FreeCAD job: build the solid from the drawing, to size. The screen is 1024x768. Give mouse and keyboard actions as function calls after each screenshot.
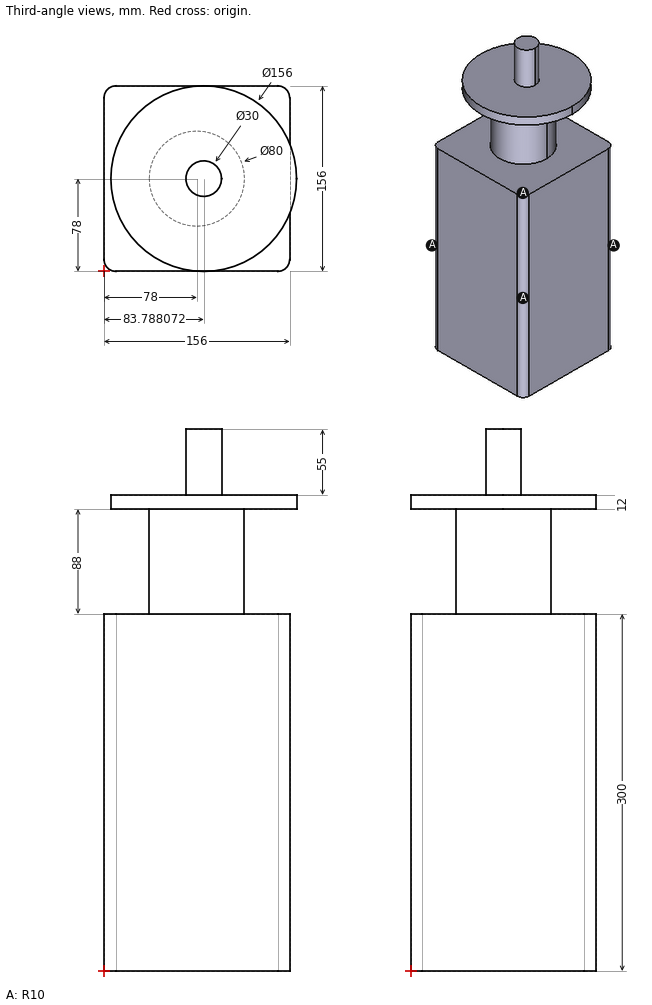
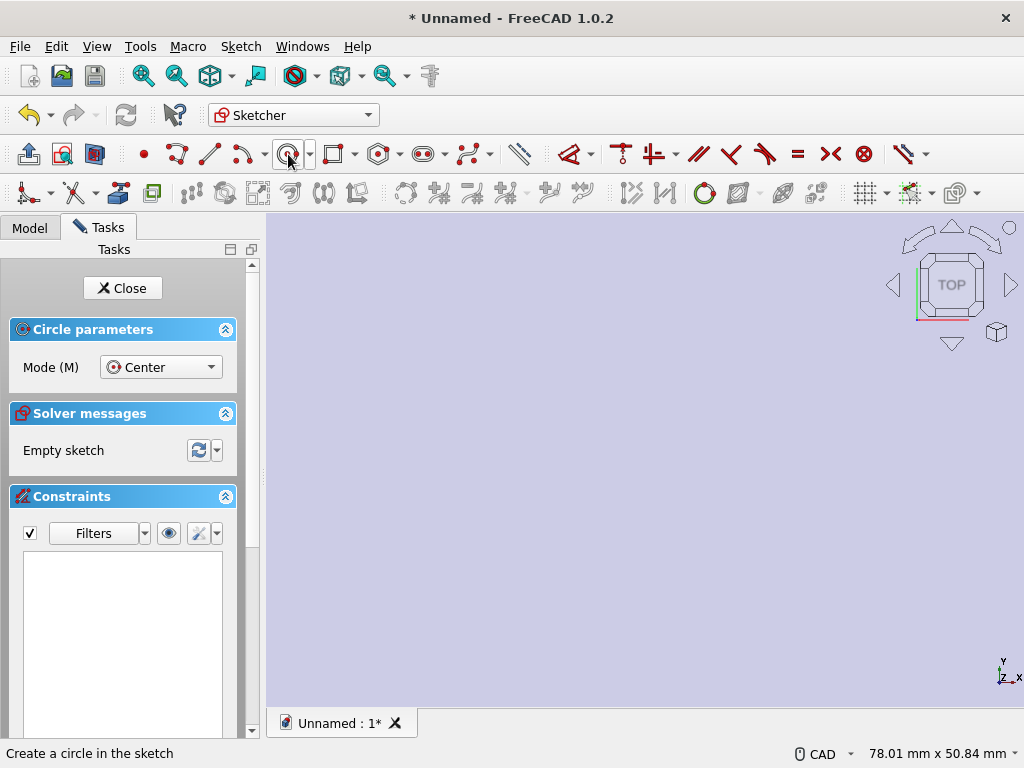
click(573, 456)
move(676, 353)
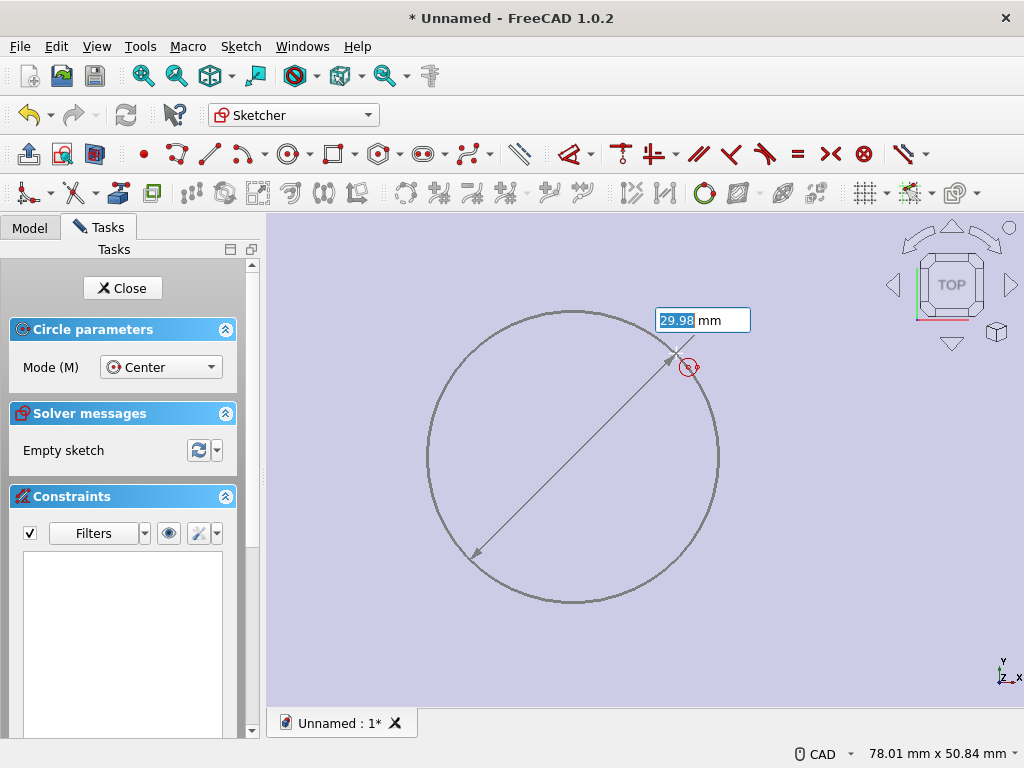
text(30)
key(Return)
key(Escape)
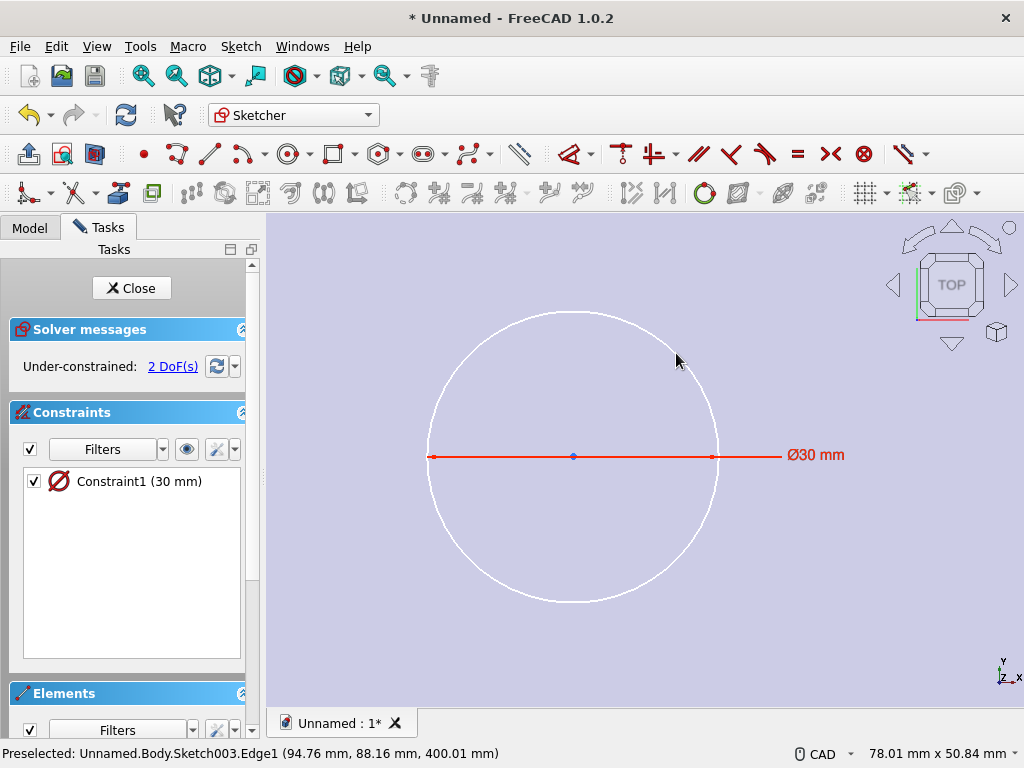
click(568, 154)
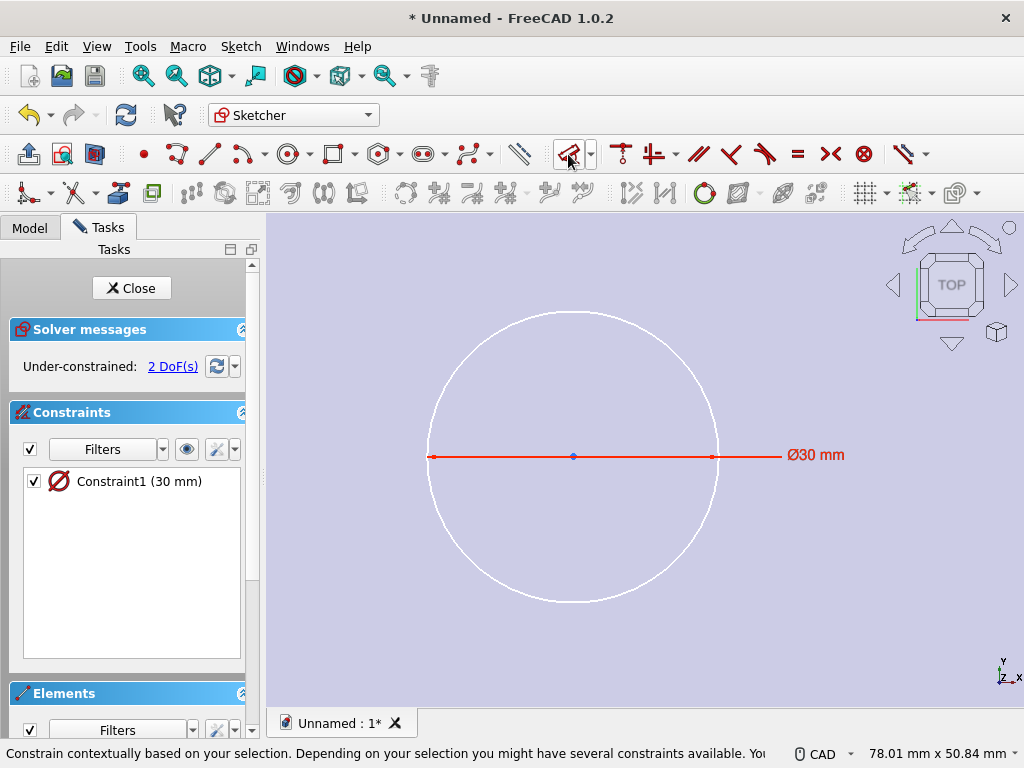
click(573, 457)
click(607, 568)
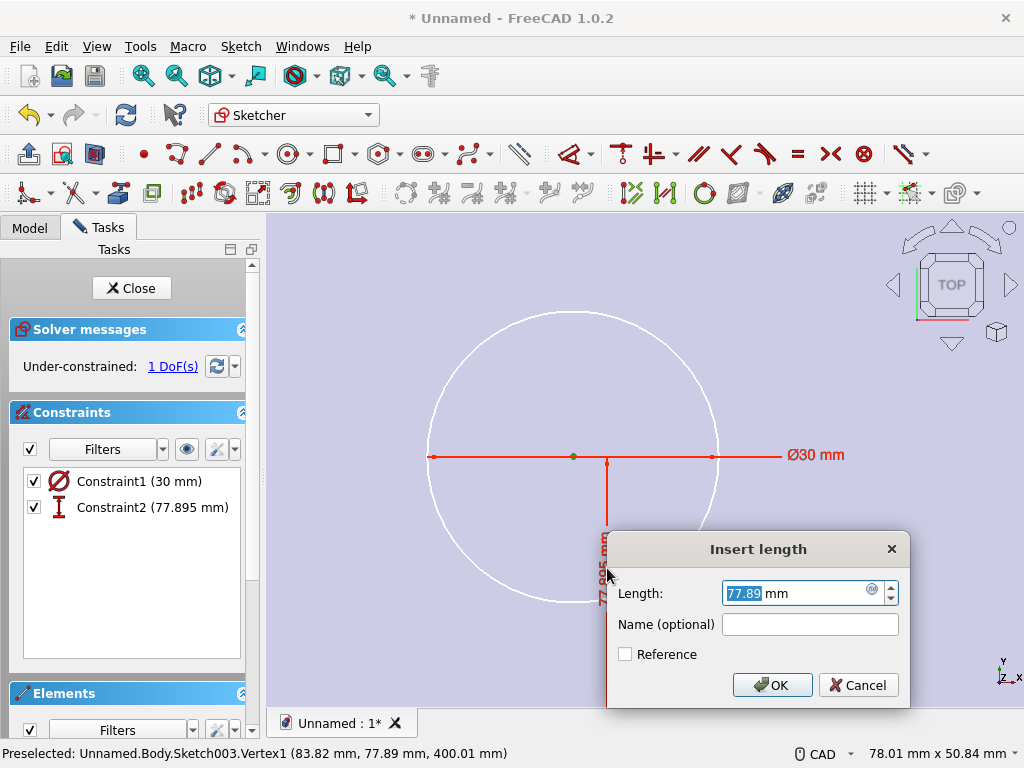
text(78)
key(Return)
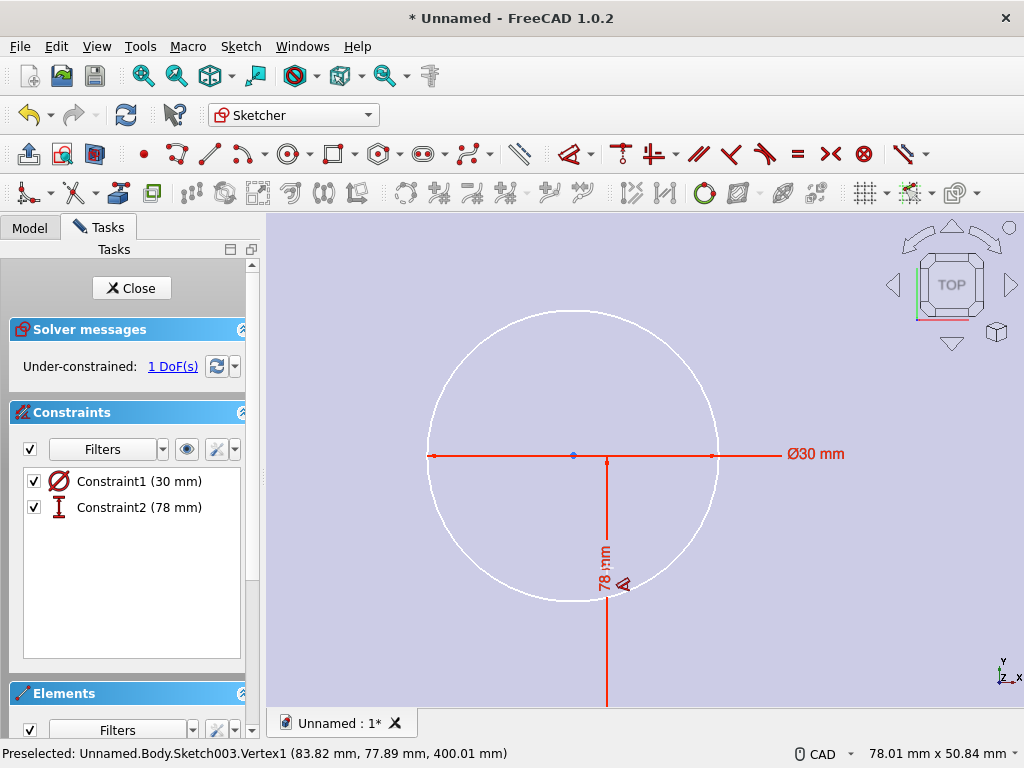
click(573, 456)
click(369, 422)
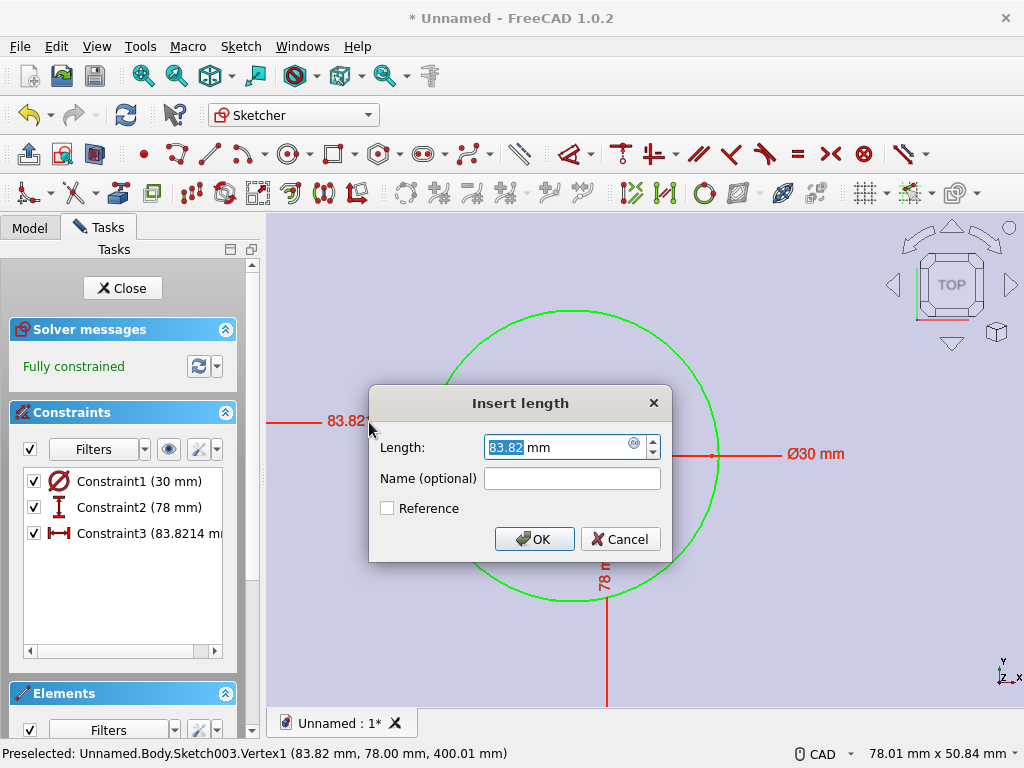
text(83.788072)
key(Return)
key(Escape)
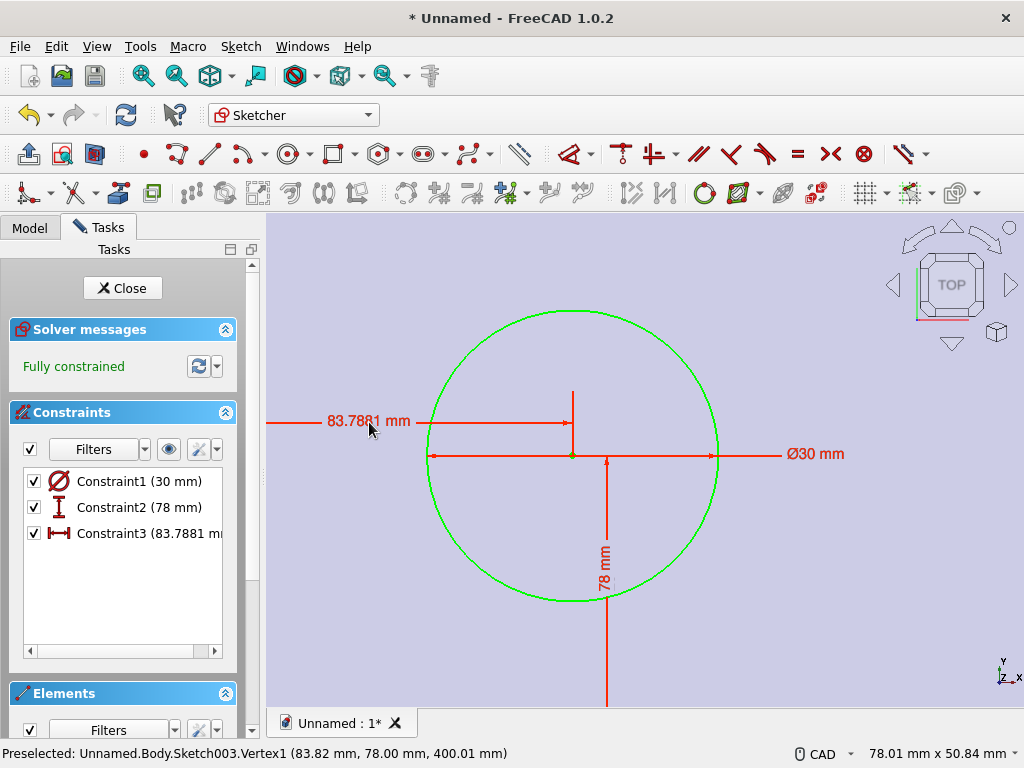
click(123, 288)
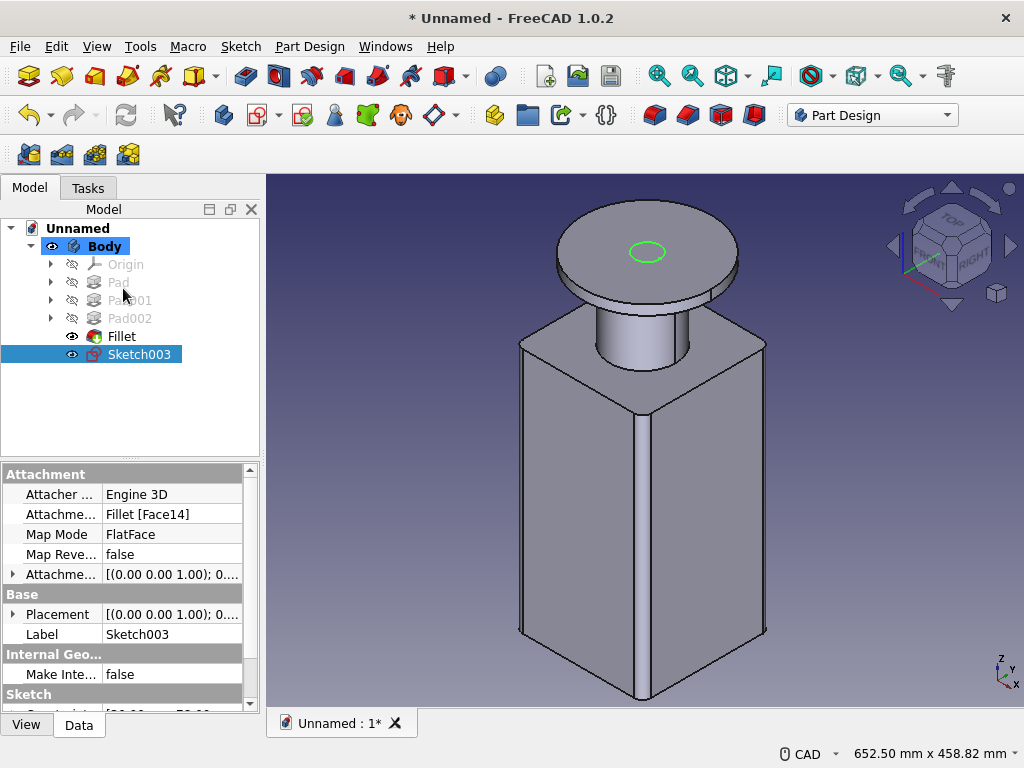
click(29, 76)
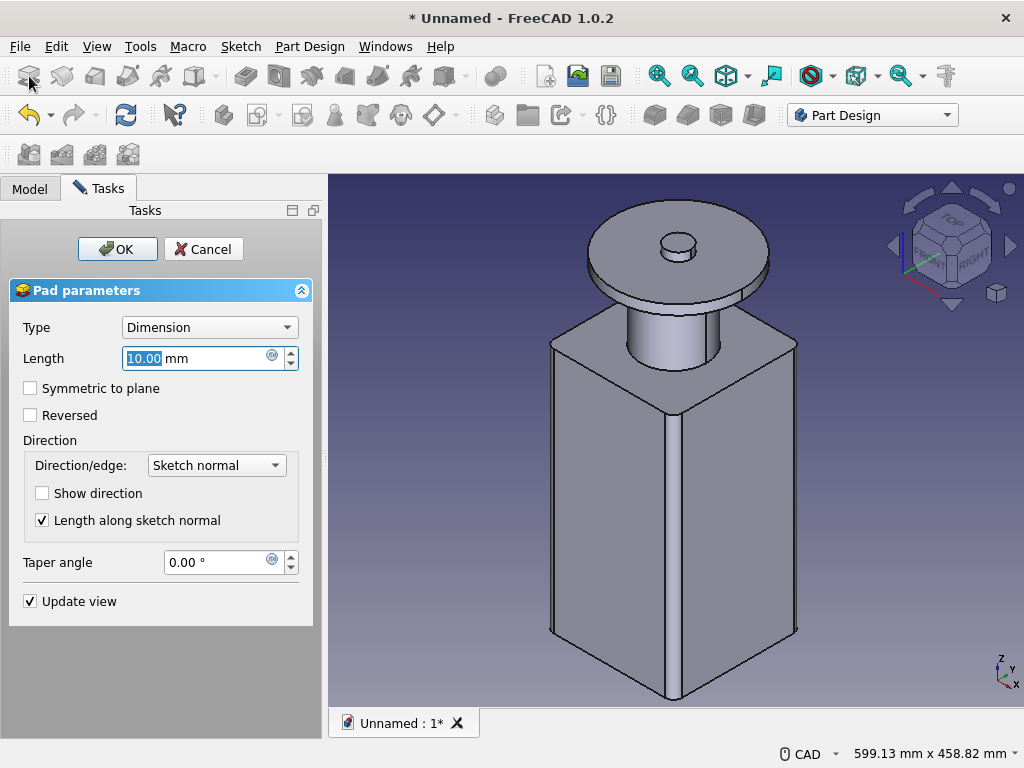
text(55)
key(Tab)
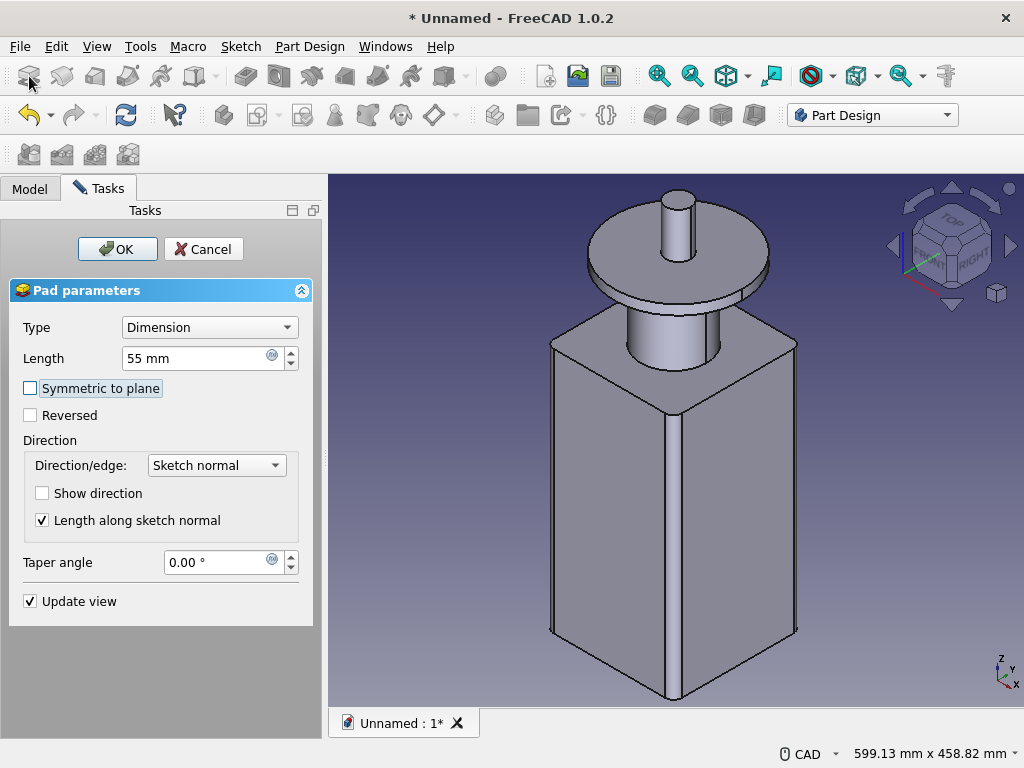
click(118, 249)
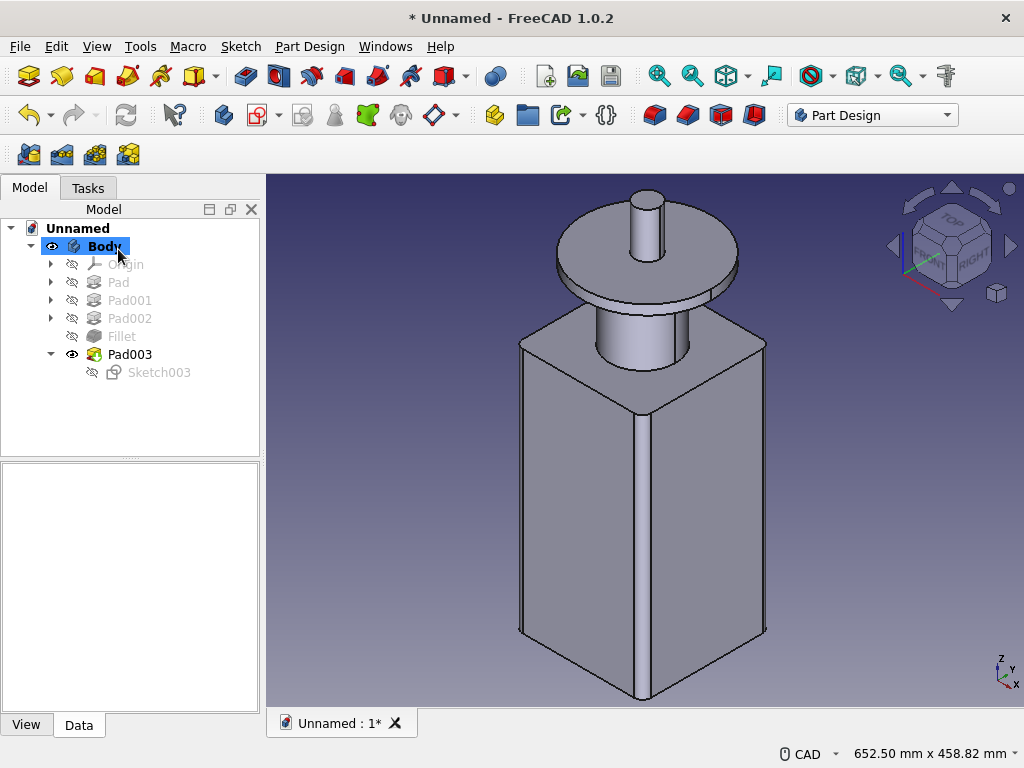
click(660, 76)